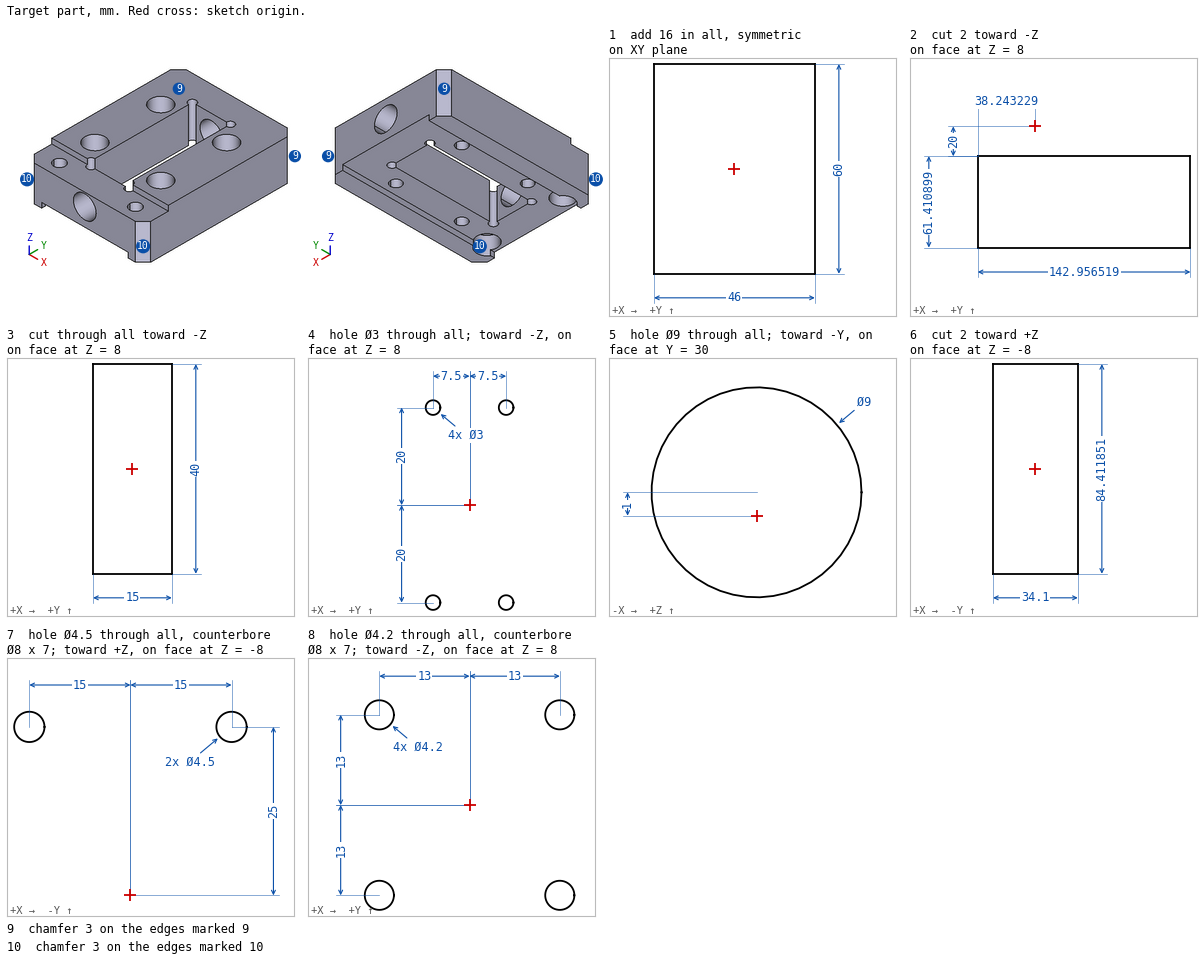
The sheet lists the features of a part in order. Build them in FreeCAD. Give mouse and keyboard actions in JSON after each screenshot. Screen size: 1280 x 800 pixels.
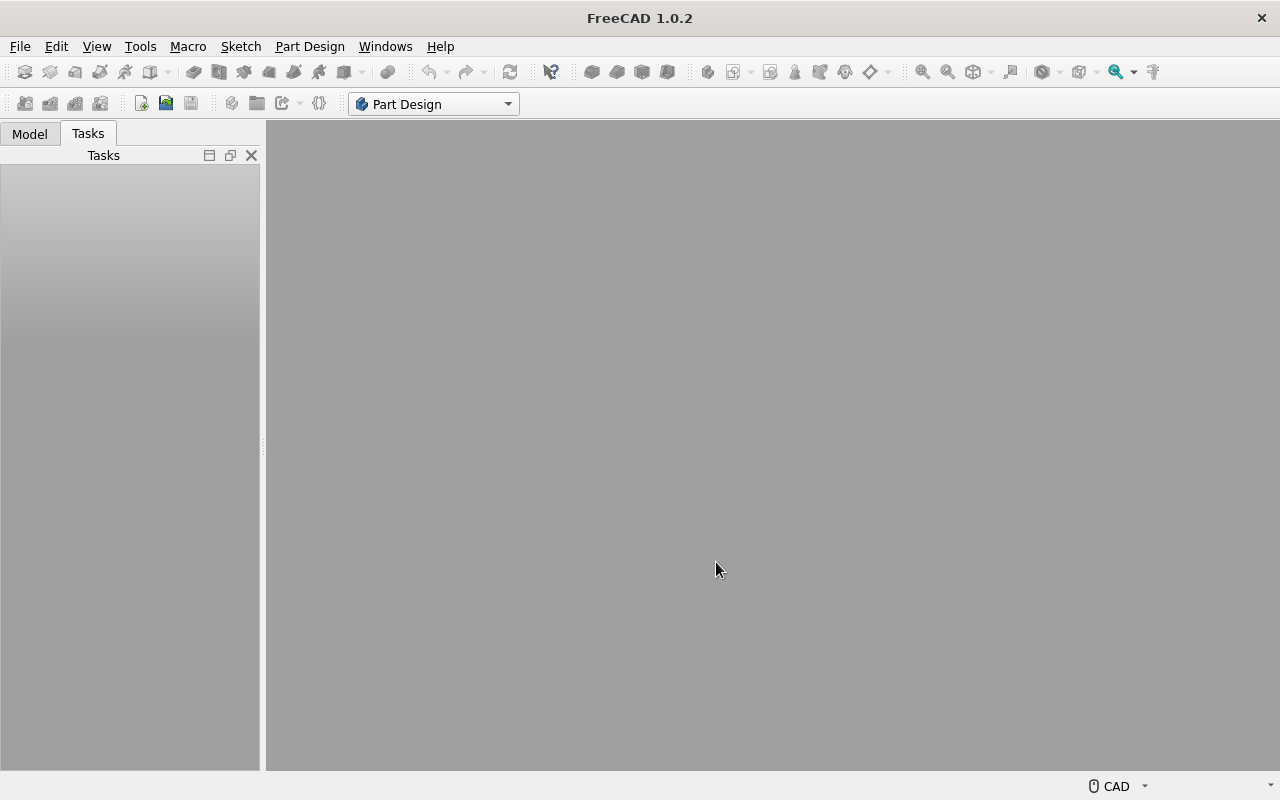
{"action": "left_click", "coordinate": [141, 104]}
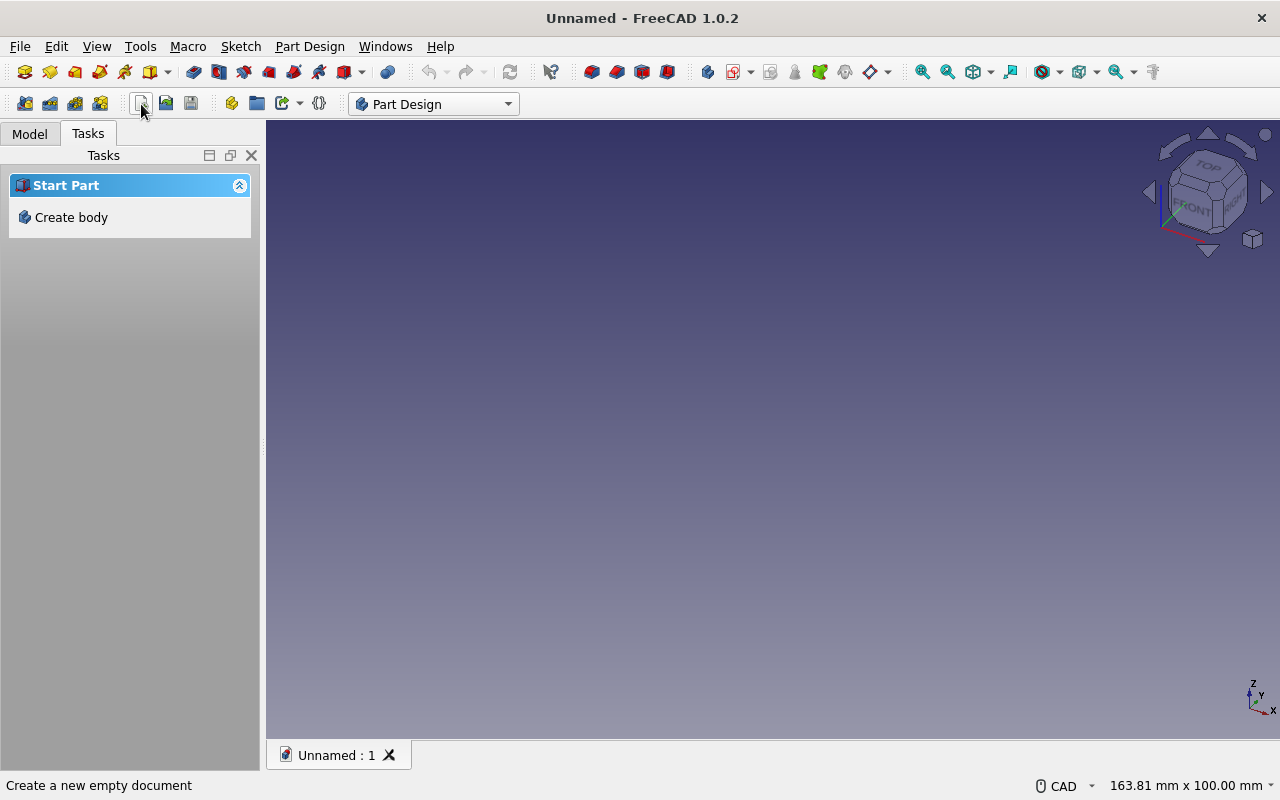
{"action": "left_click", "coordinate": [732, 72]}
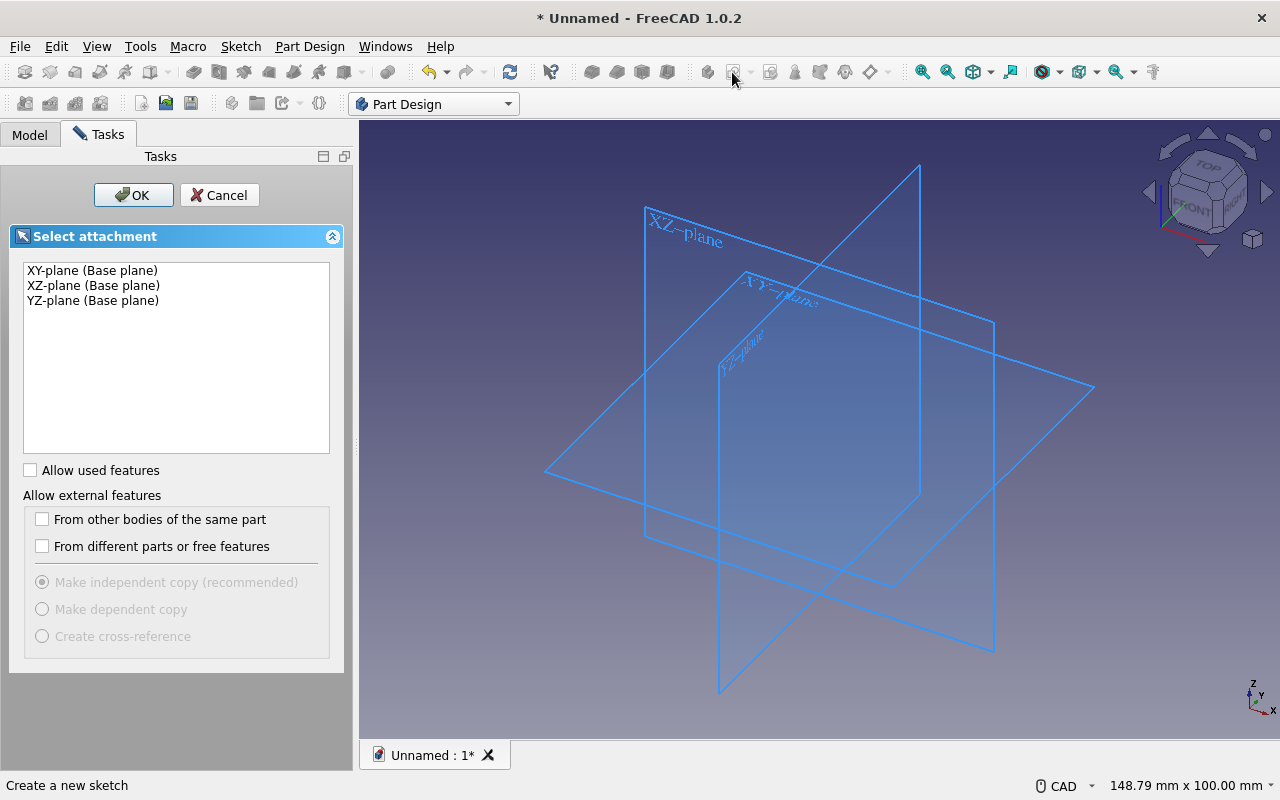
{"action": "left_click", "coordinate": [84, 270]}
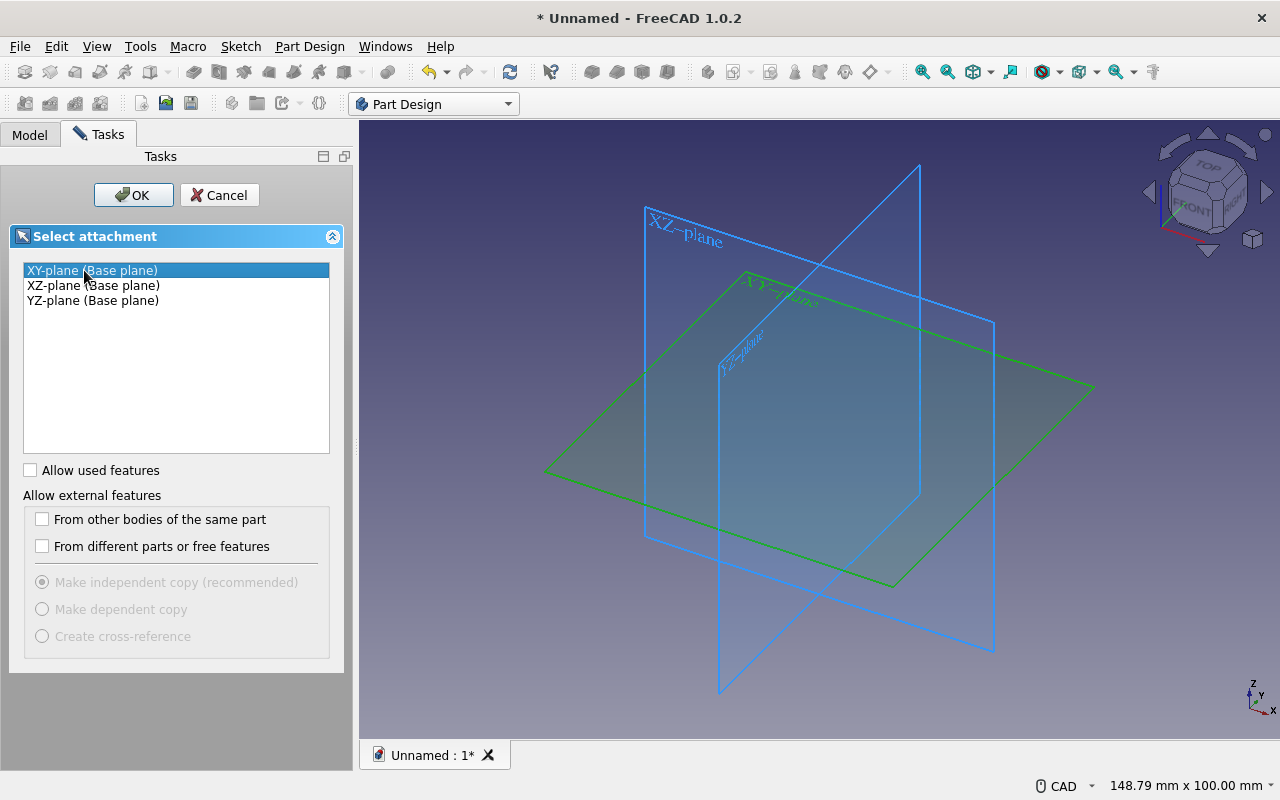
{"action": "left_click", "coordinate": [134, 195]}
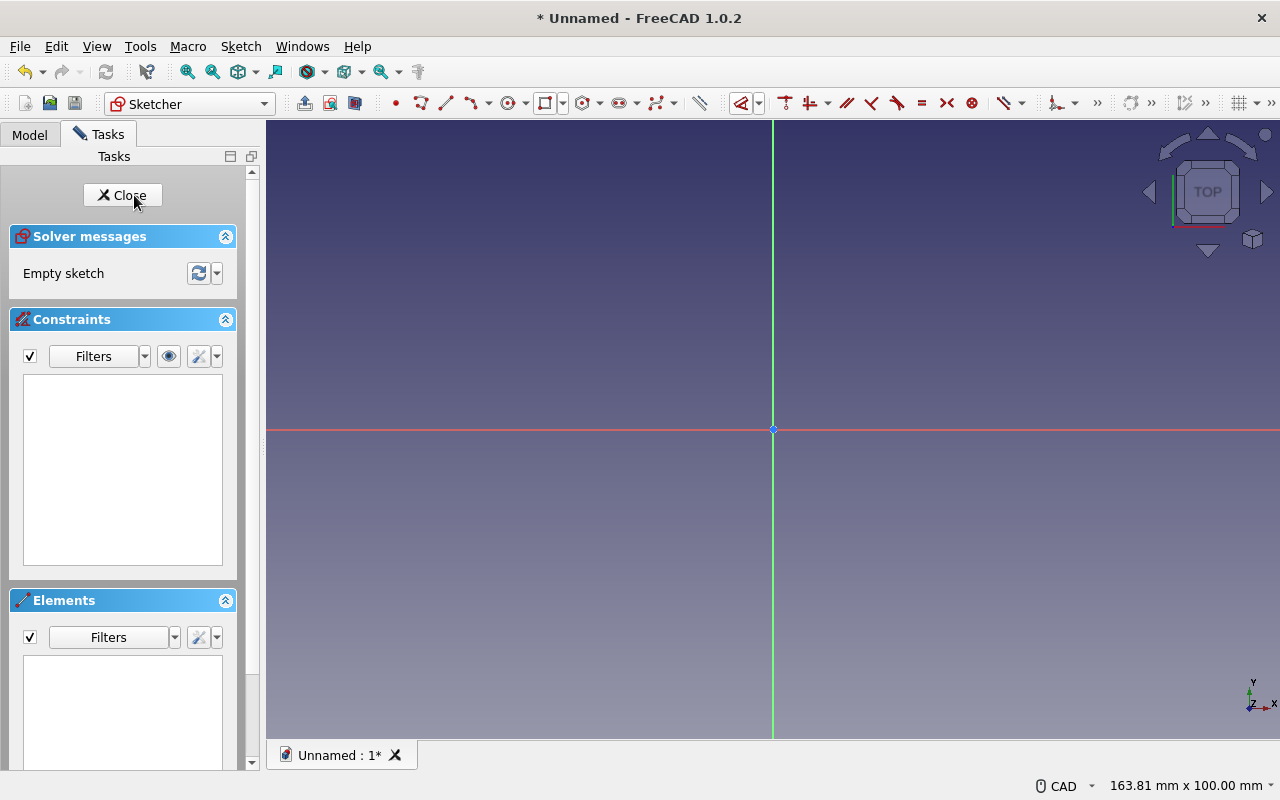
{"action": "key", "text": "g v"}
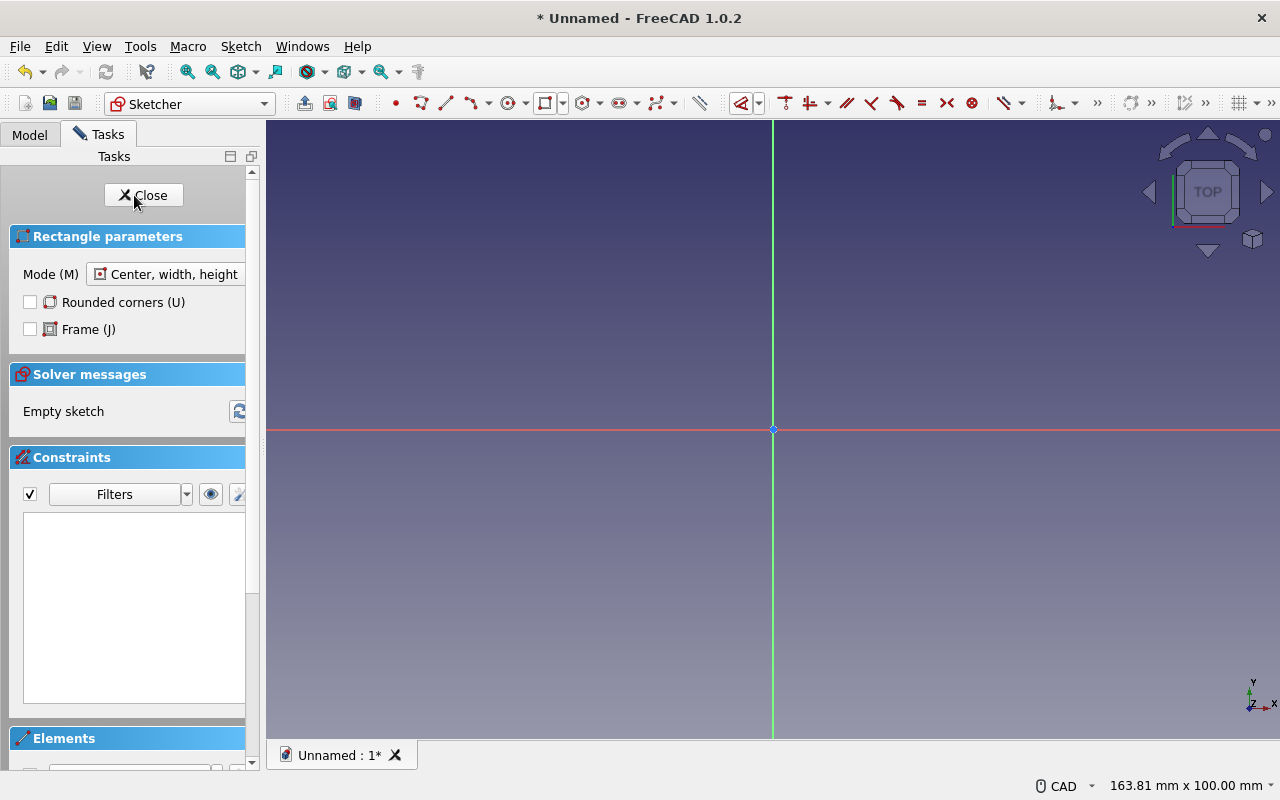
{"action": "left_click", "coordinate": [773, 430]}
{"action": "left_click", "coordinate": [915, 244]}
{"action": "key", "text": "Escape"}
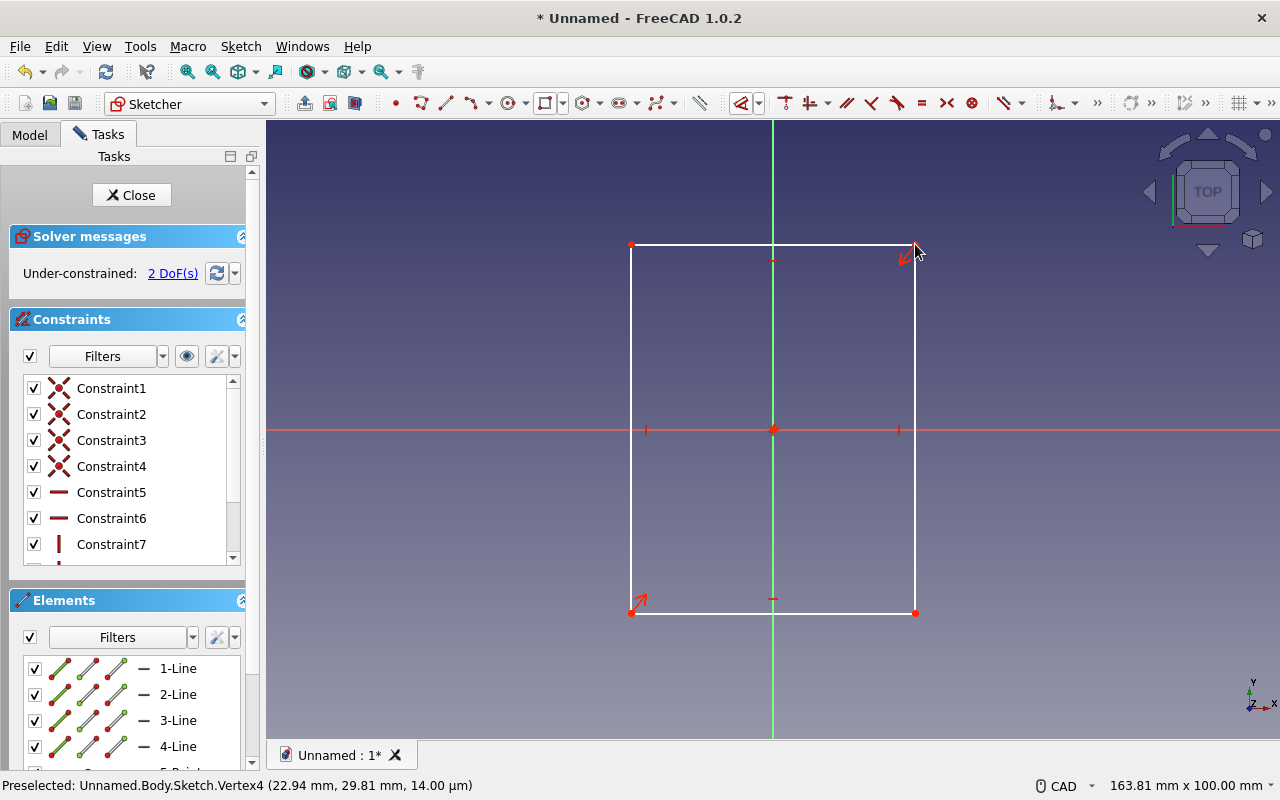
{"action": "left_click", "coordinate": [740, 104]}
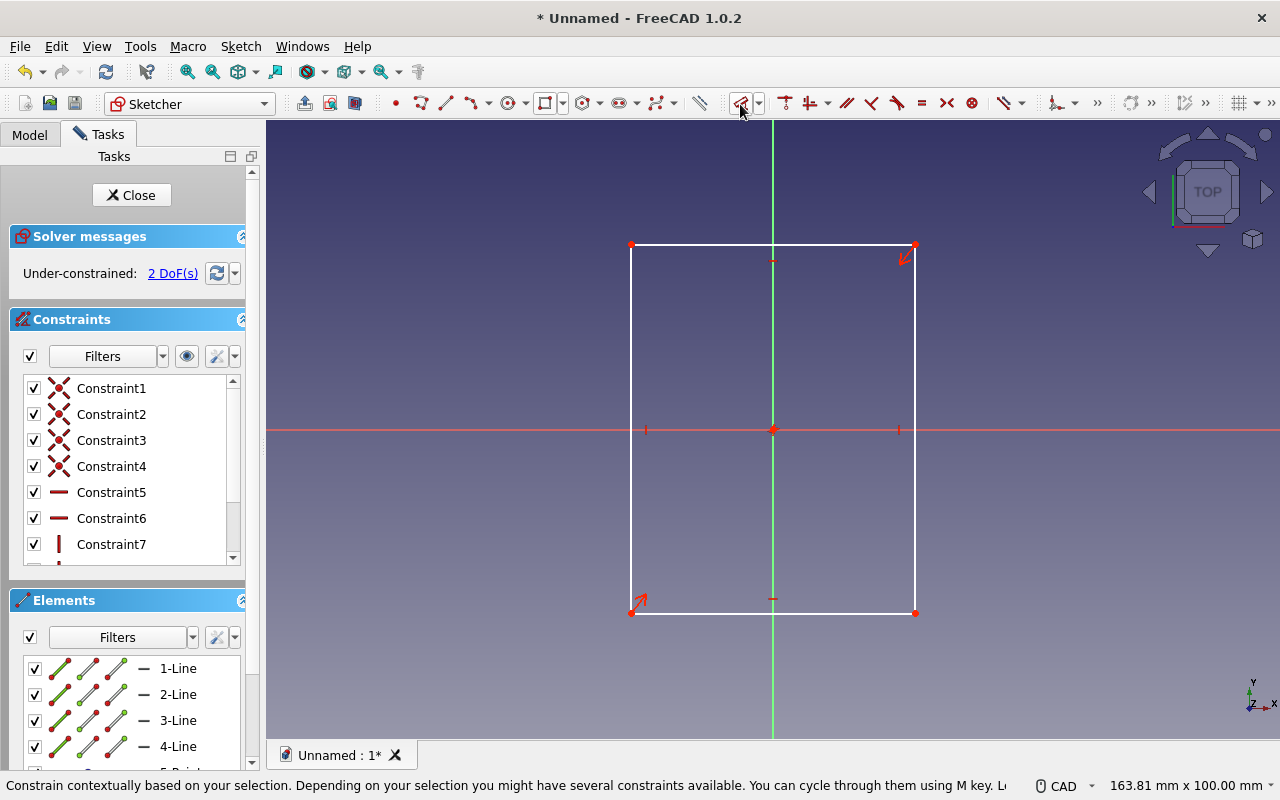
{"action": "left_click", "coordinate": [716, 614]}
{"action": "left_click", "coordinate": [708, 648]}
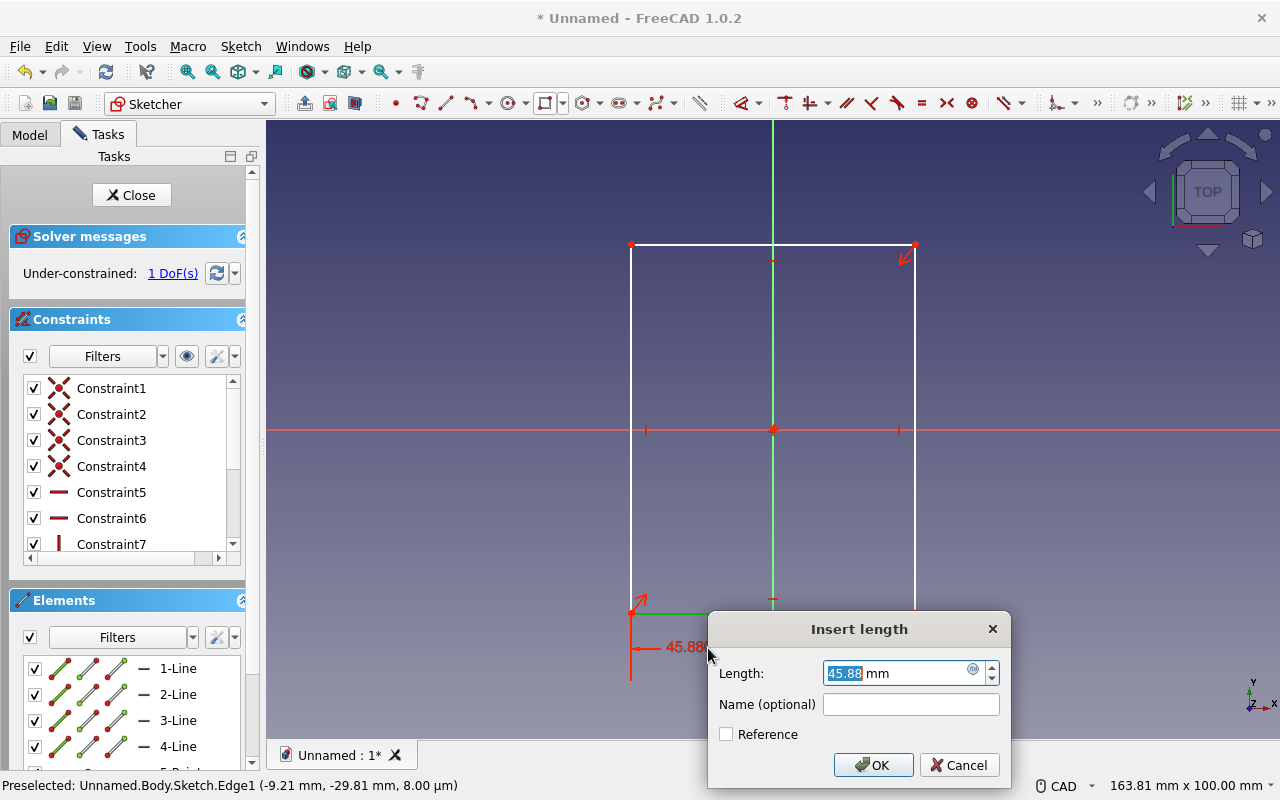
{"action": "type", "text": "46"}
{"action": "key", "text": "Return"}